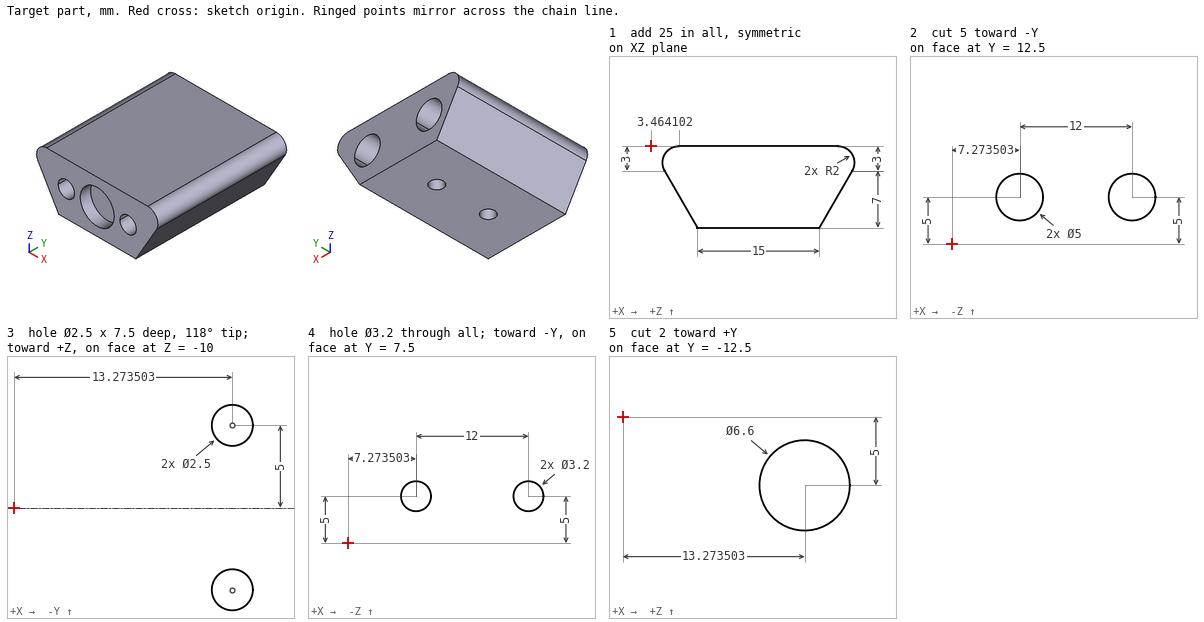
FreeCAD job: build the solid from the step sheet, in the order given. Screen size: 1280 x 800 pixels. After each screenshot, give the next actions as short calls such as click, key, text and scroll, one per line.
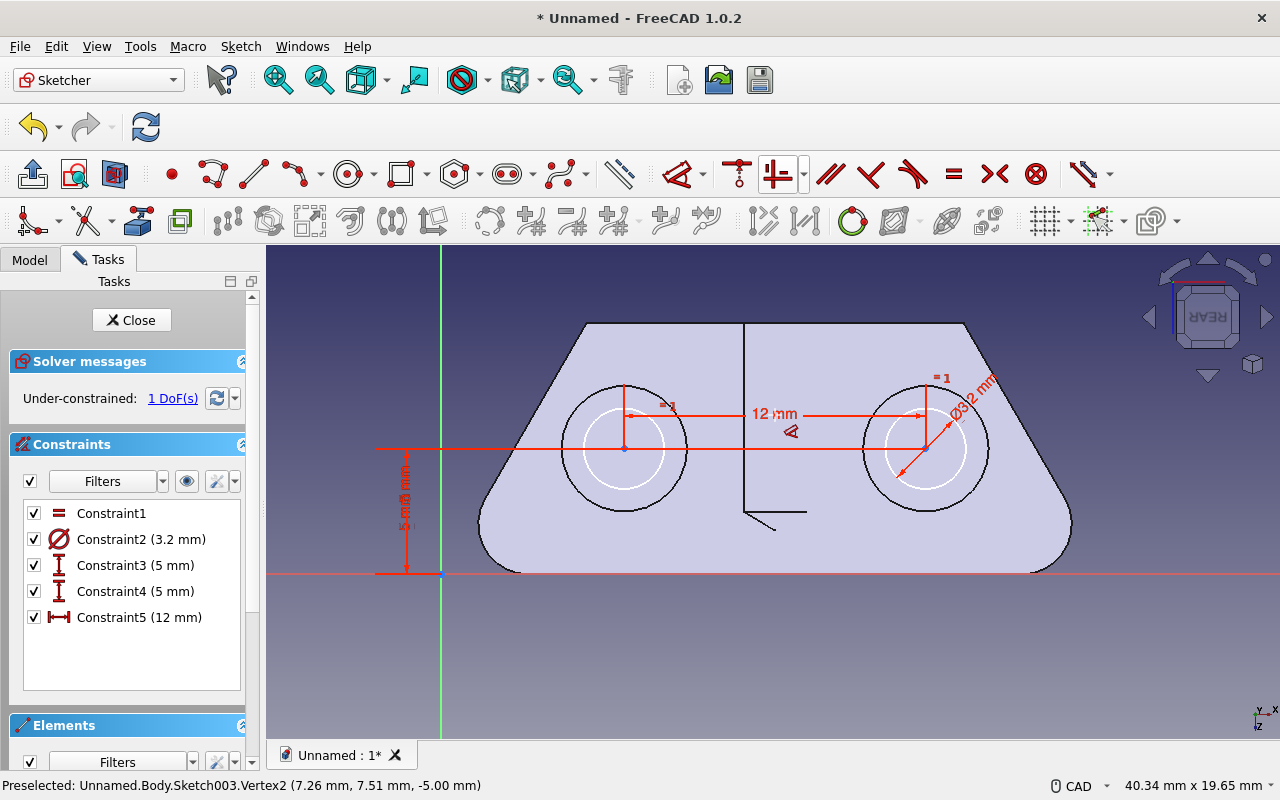
click(624, 449)
click(533, 608)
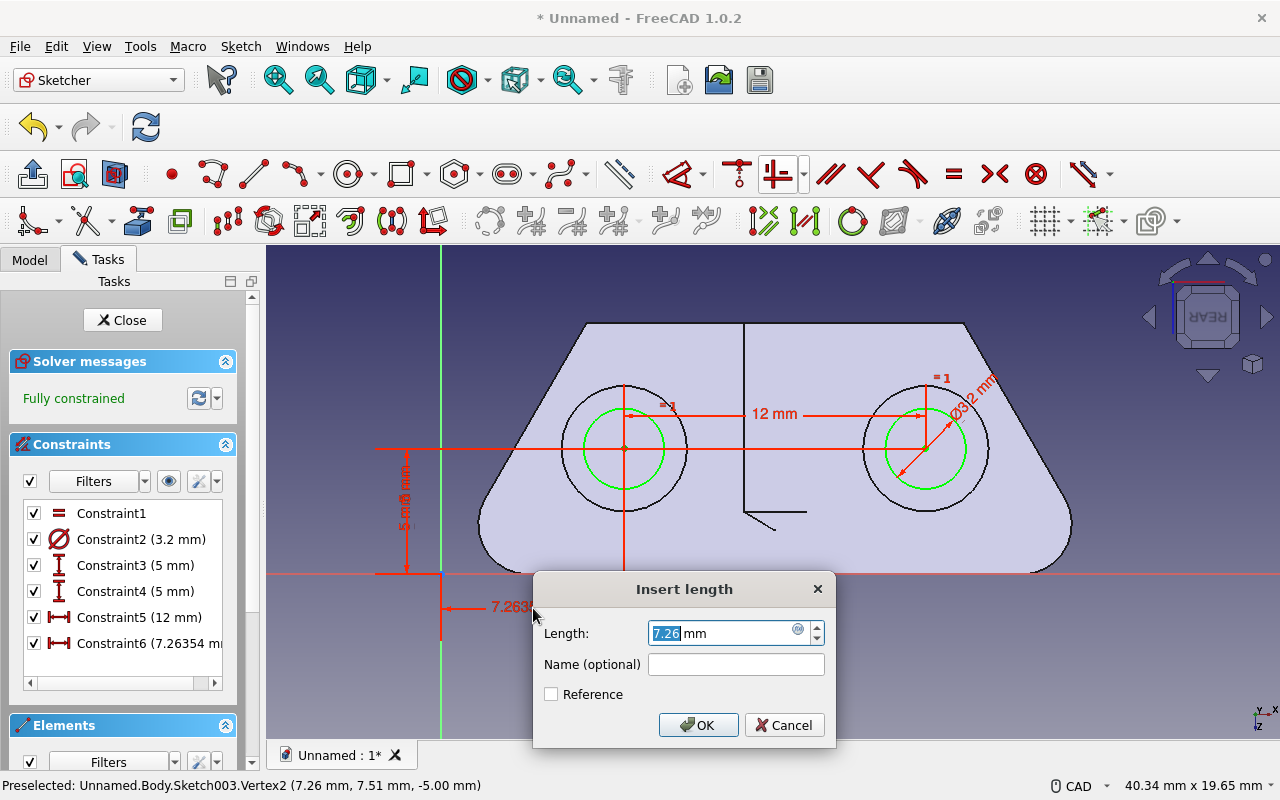
text(7.273503)
key(Return)
key(Escape)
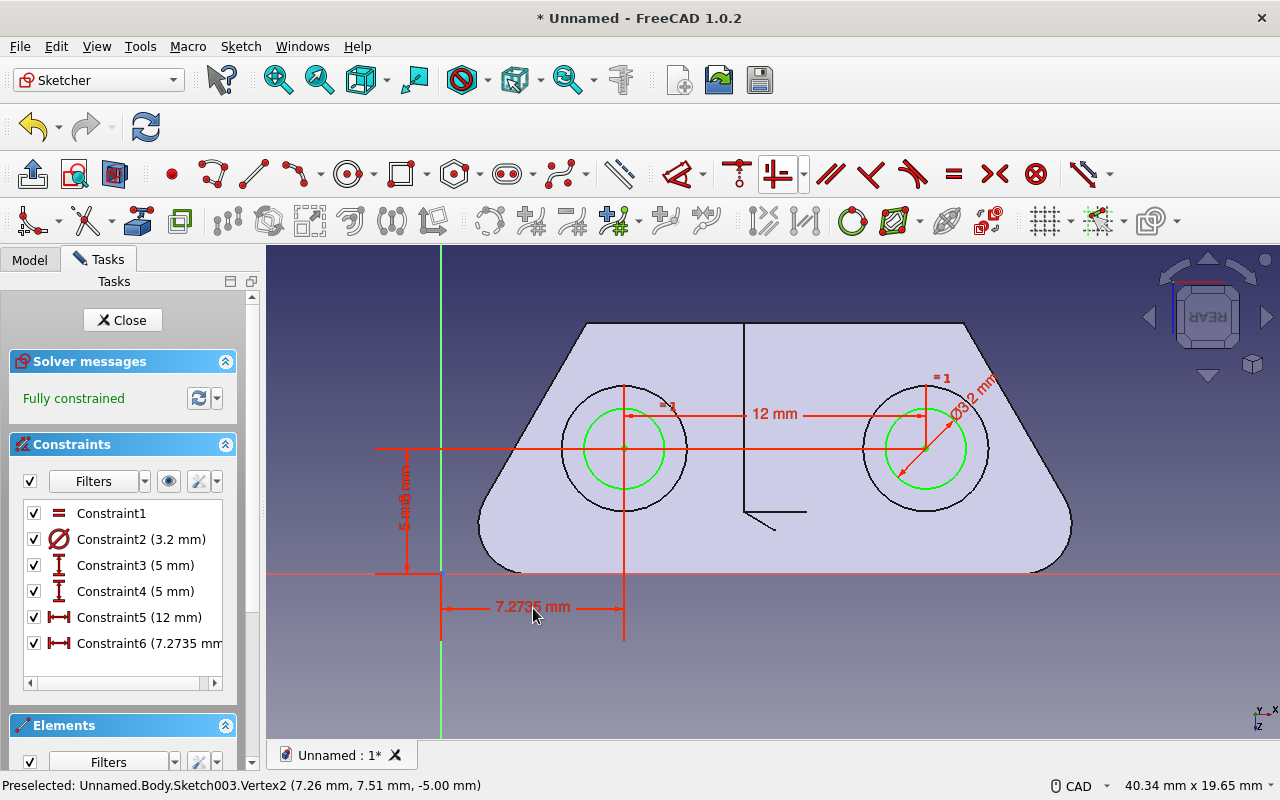
click(123, 320)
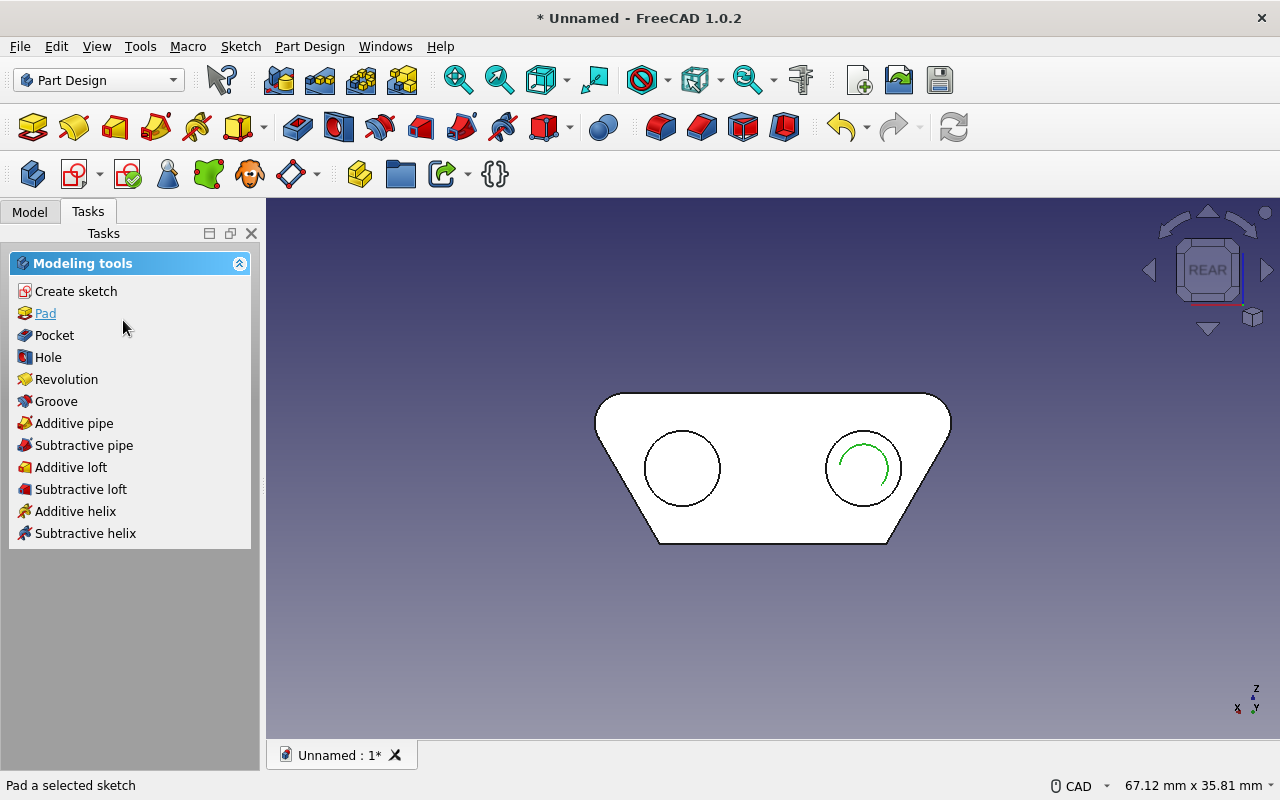
click(339, 128)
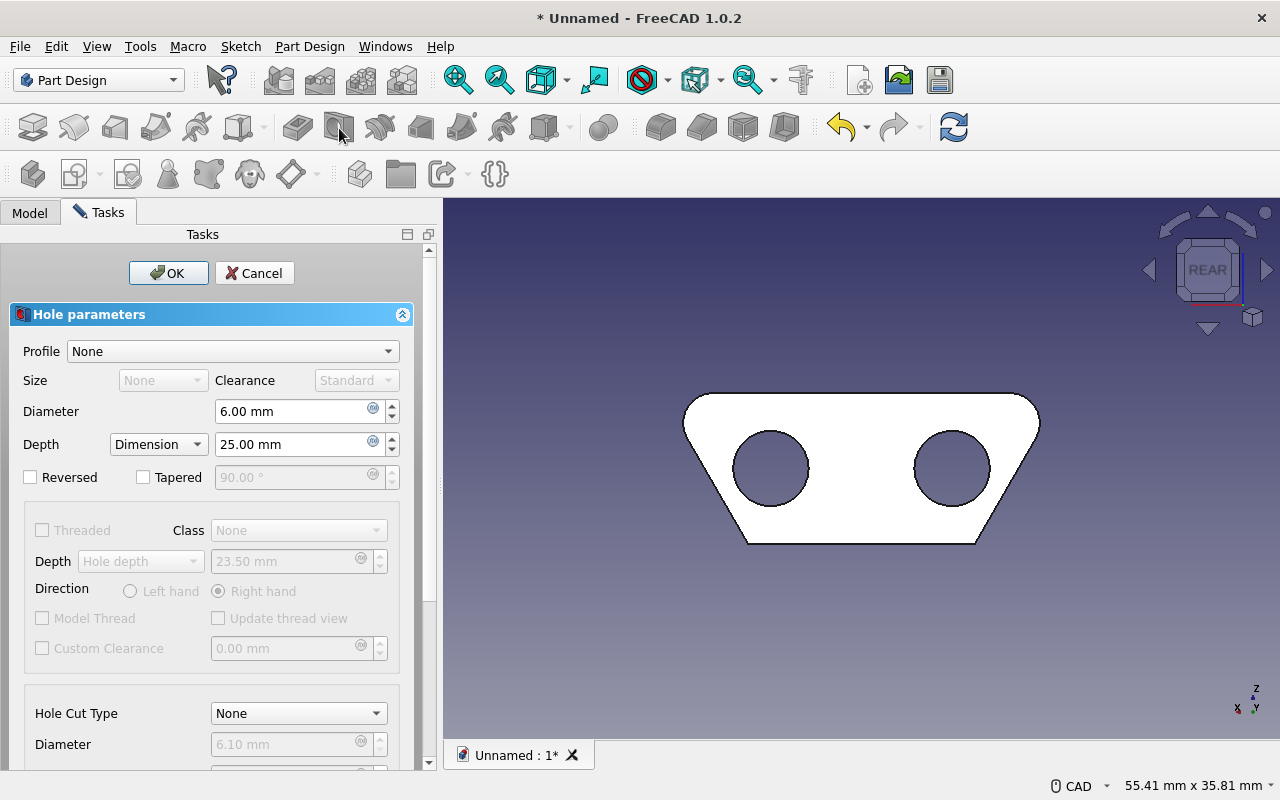
triple_click(300, 412)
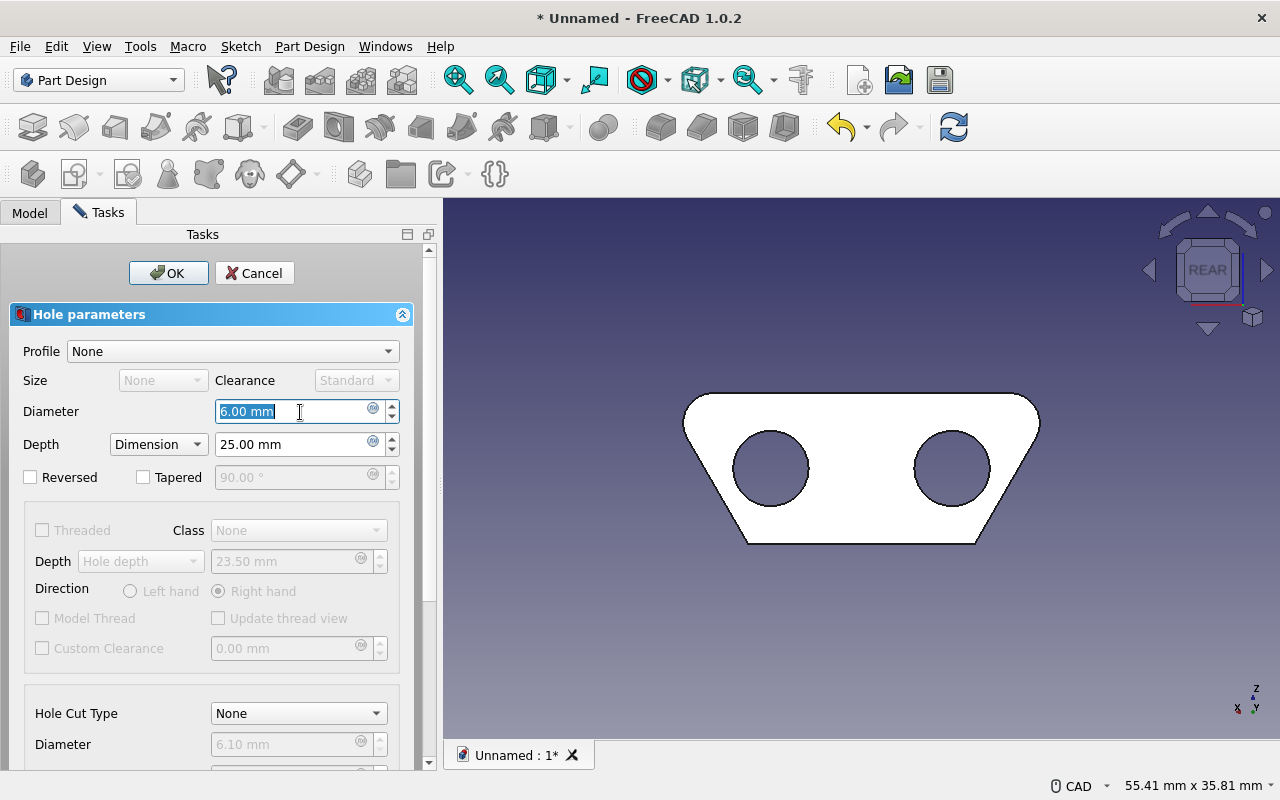
text(3.2)
key(Tab)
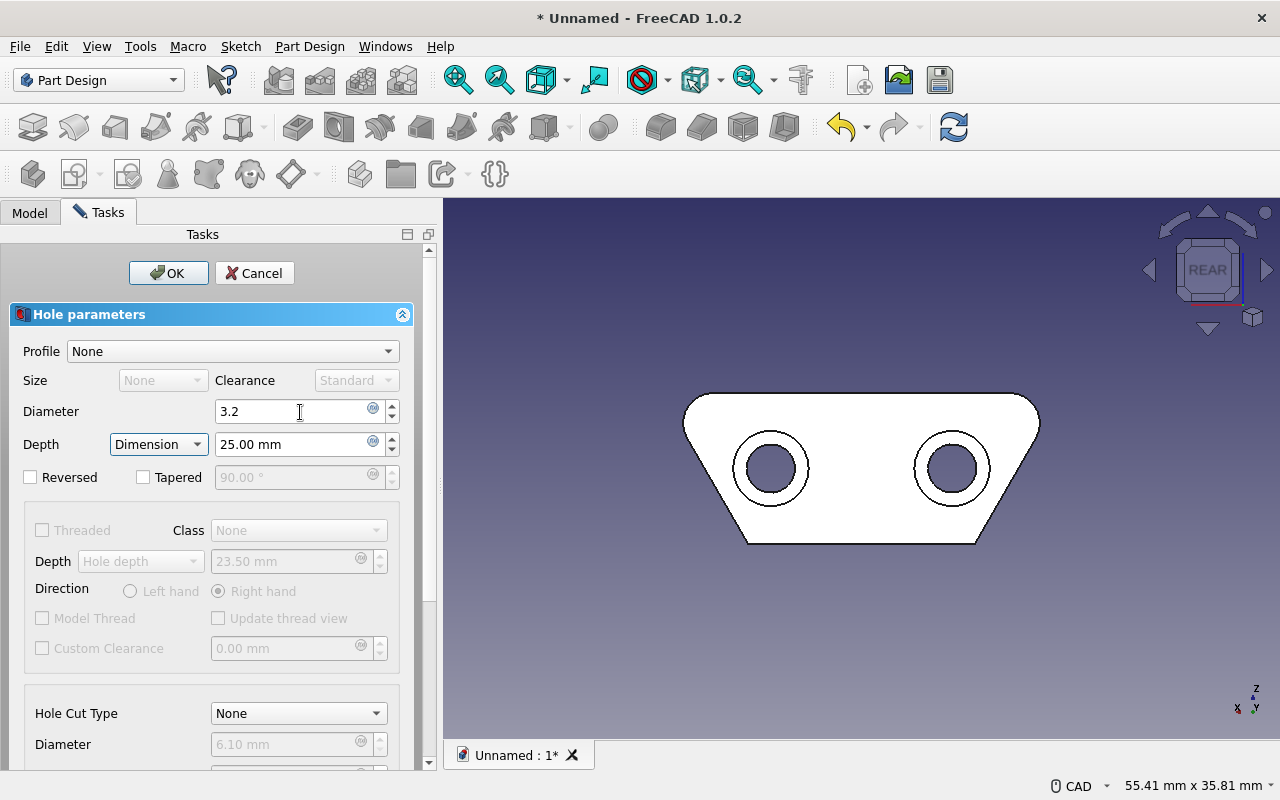
click(160, 444)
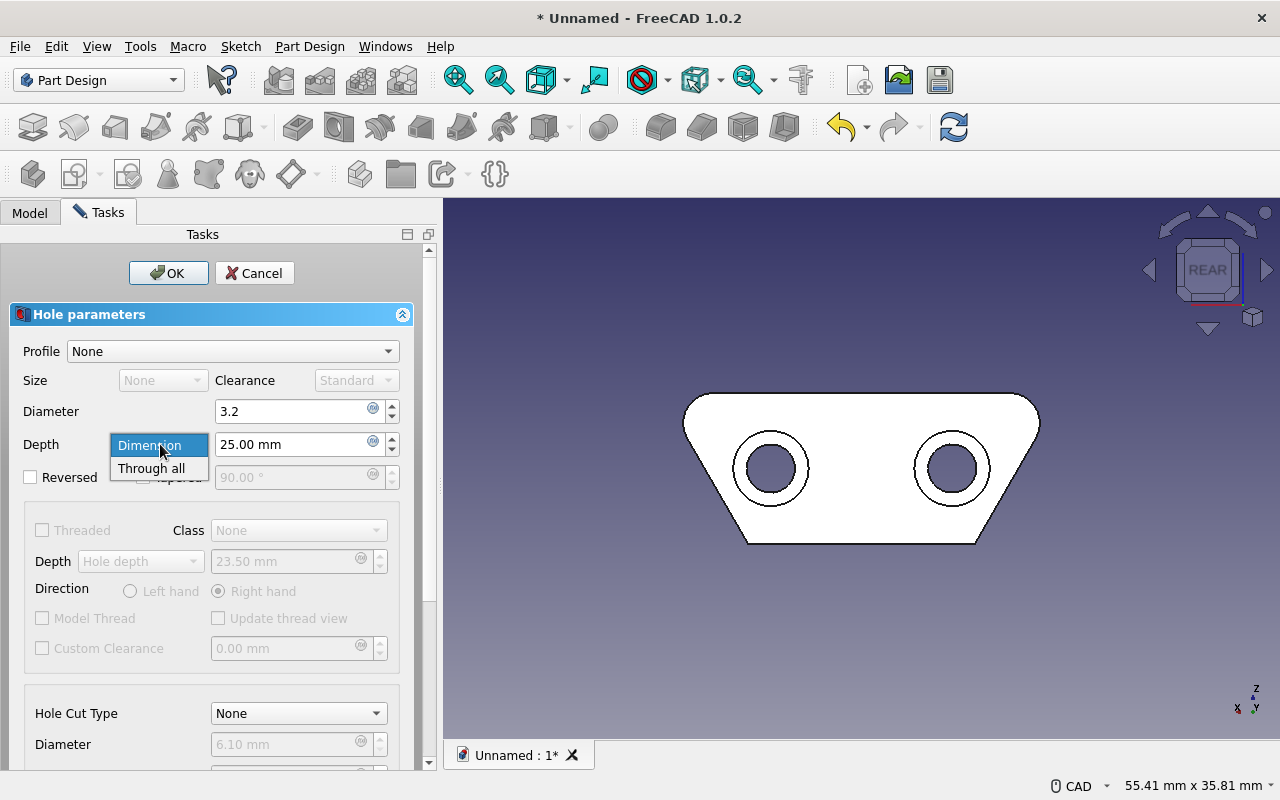
click(158, 468)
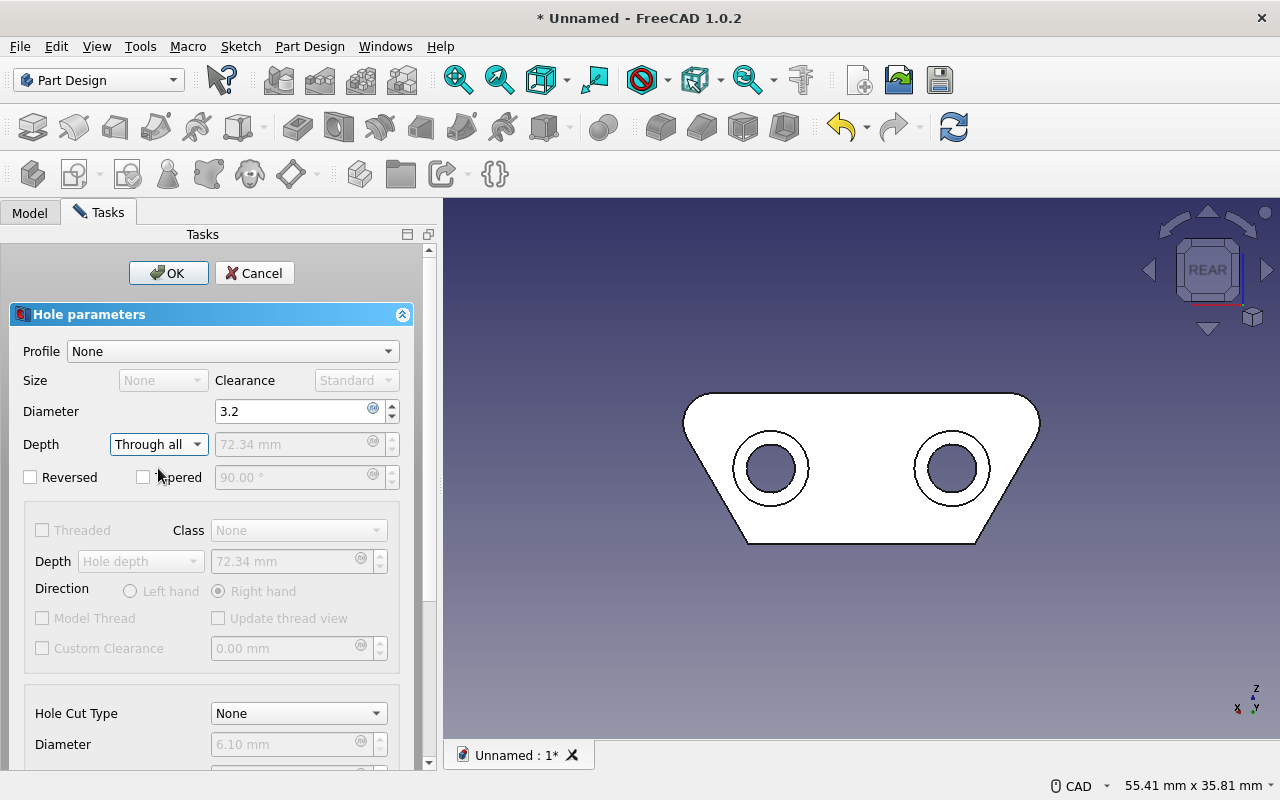
click(169, 273)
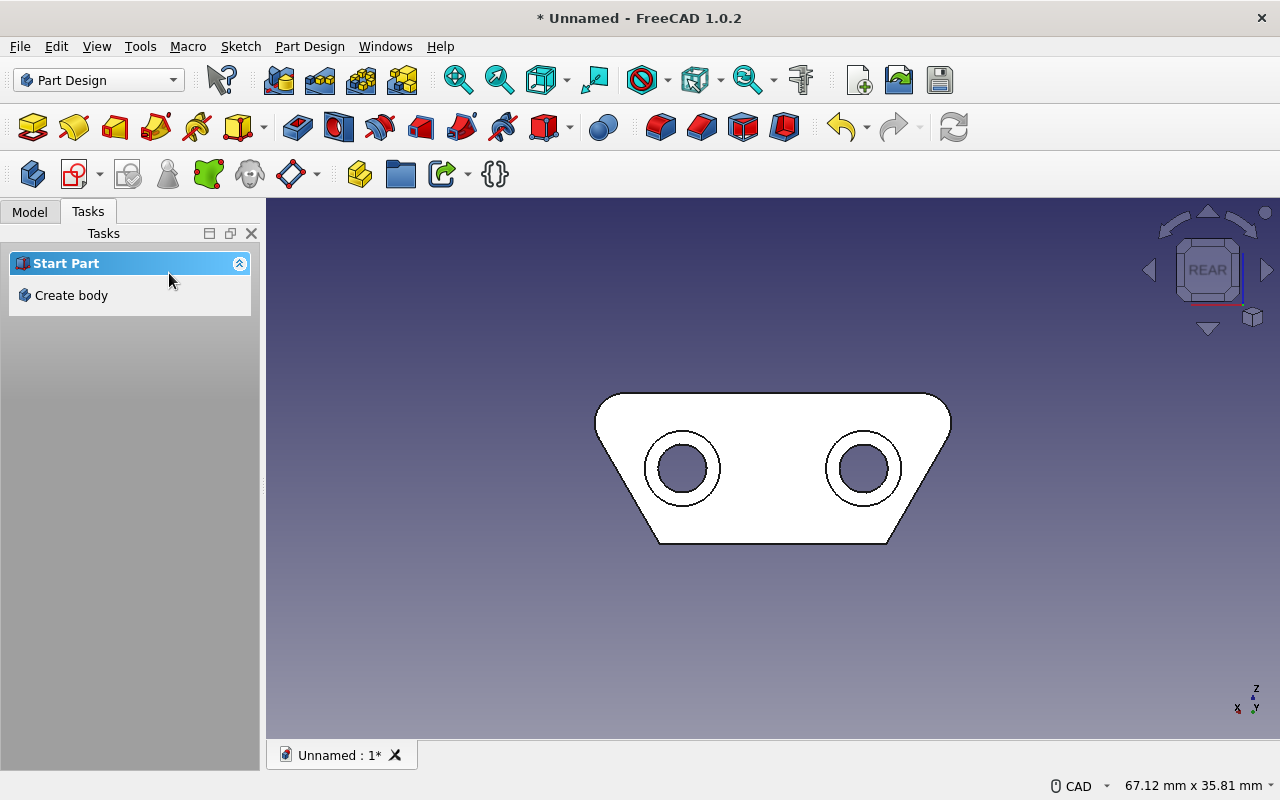
click(459, 80)